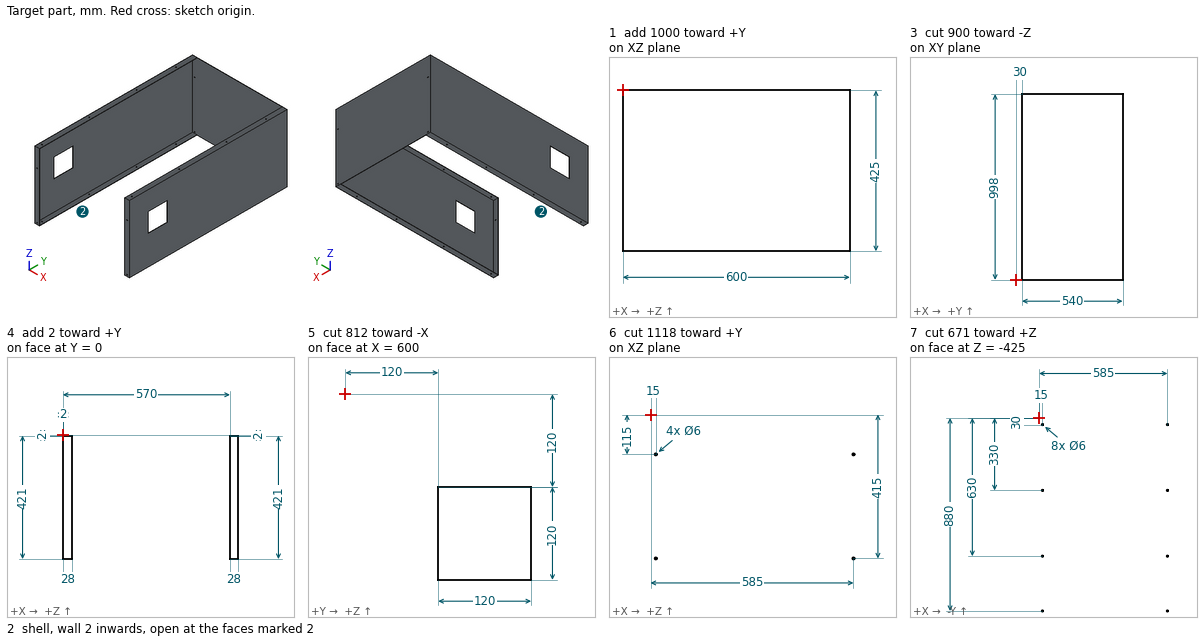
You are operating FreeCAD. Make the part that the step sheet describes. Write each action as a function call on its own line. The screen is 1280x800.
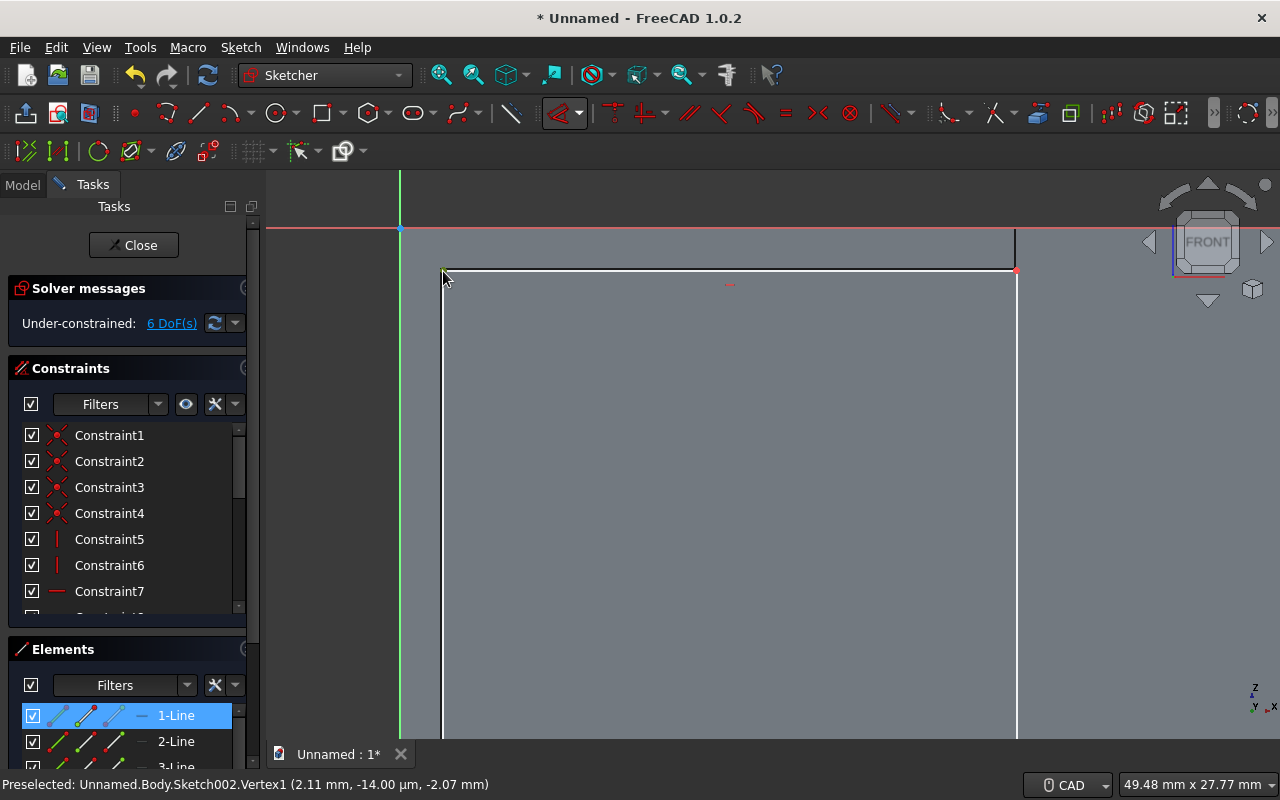
click(582, 114)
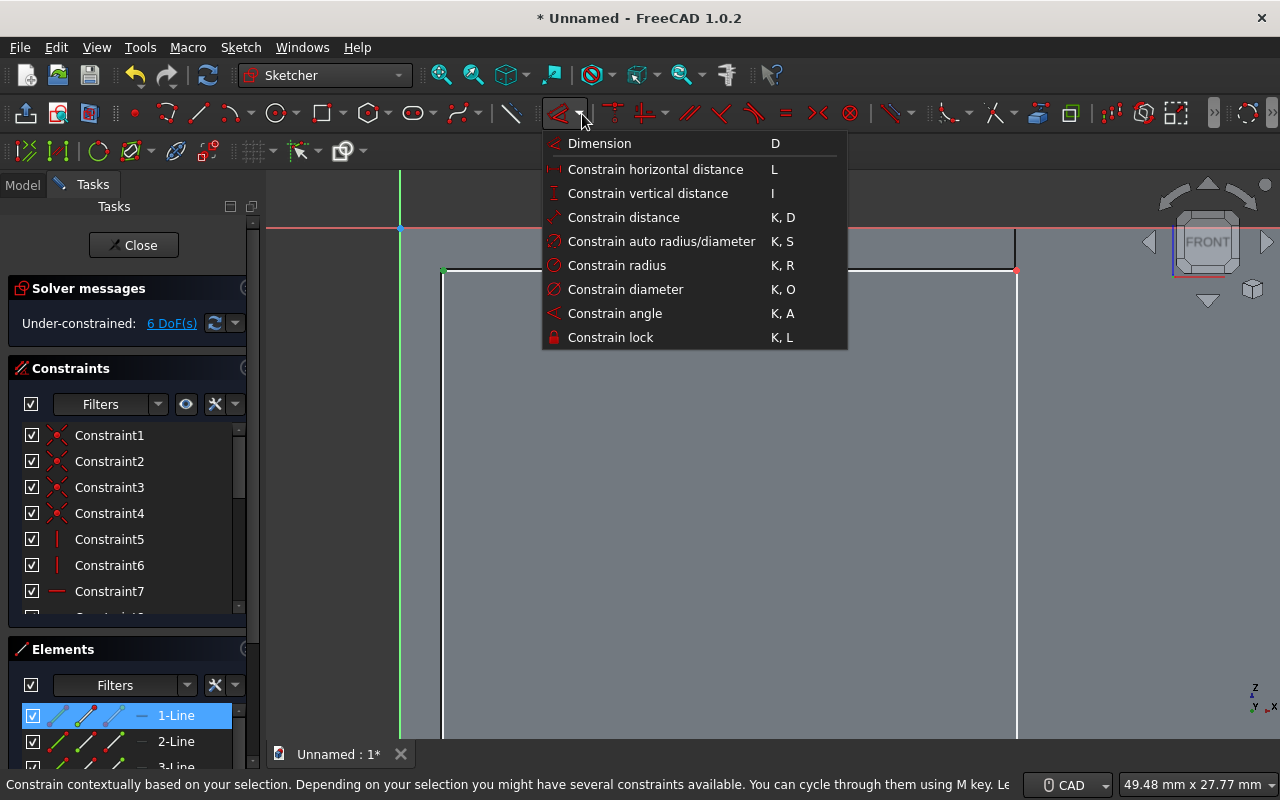
click(695, 169)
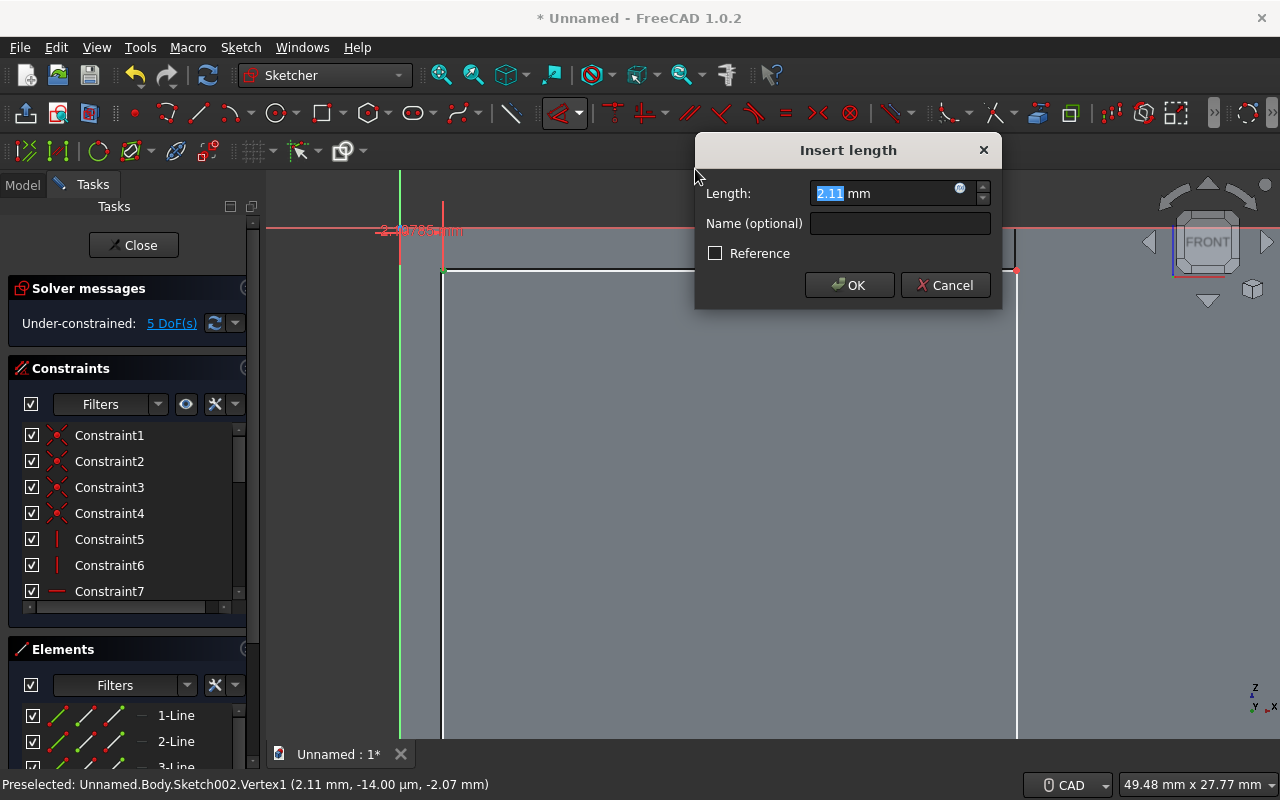
text(2)
key(Return)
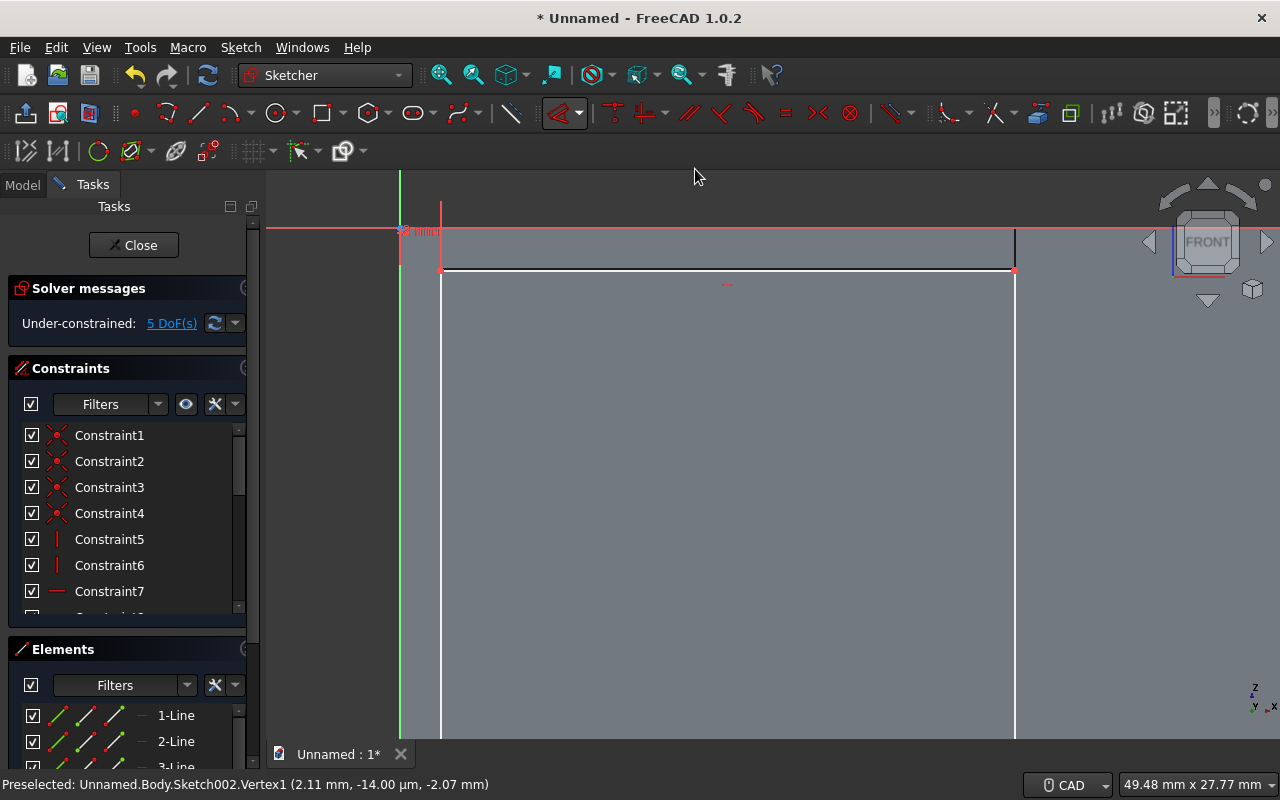
click(441, 271)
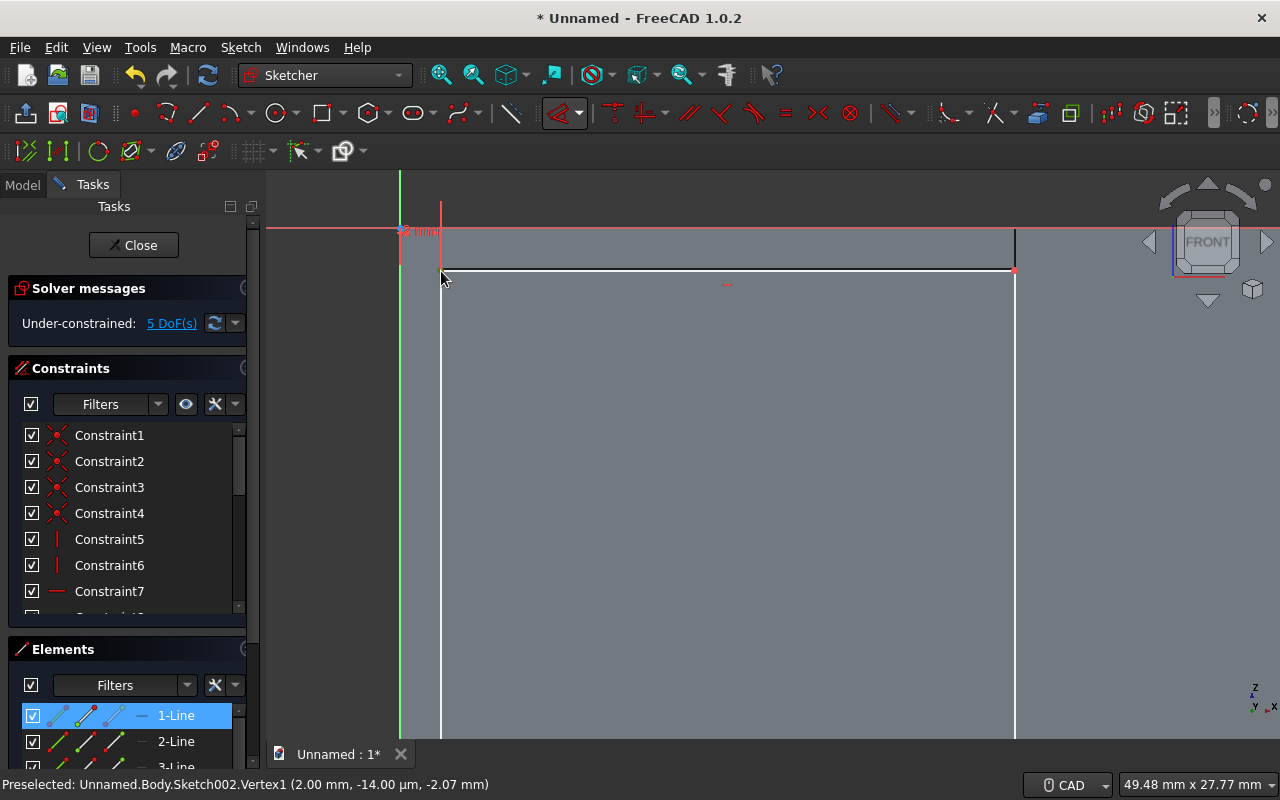
click(582, 114)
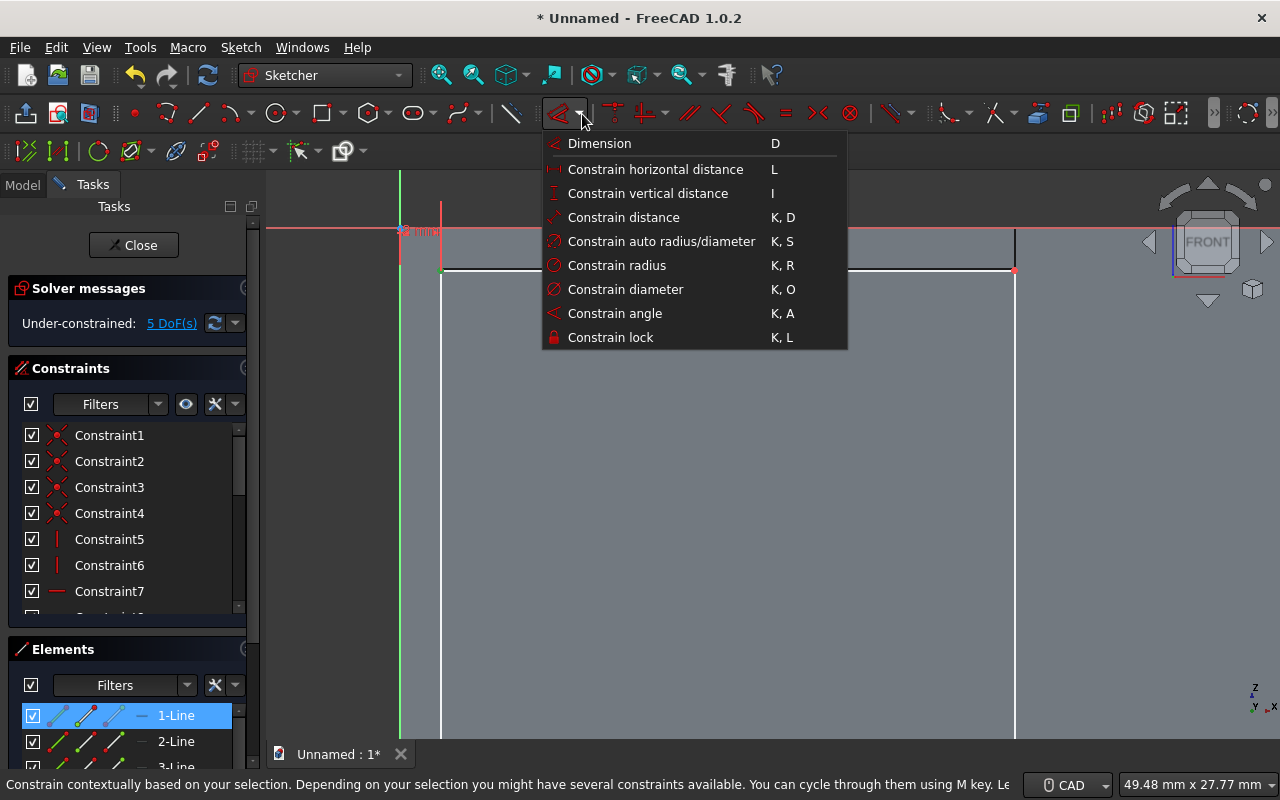
click(695, 193)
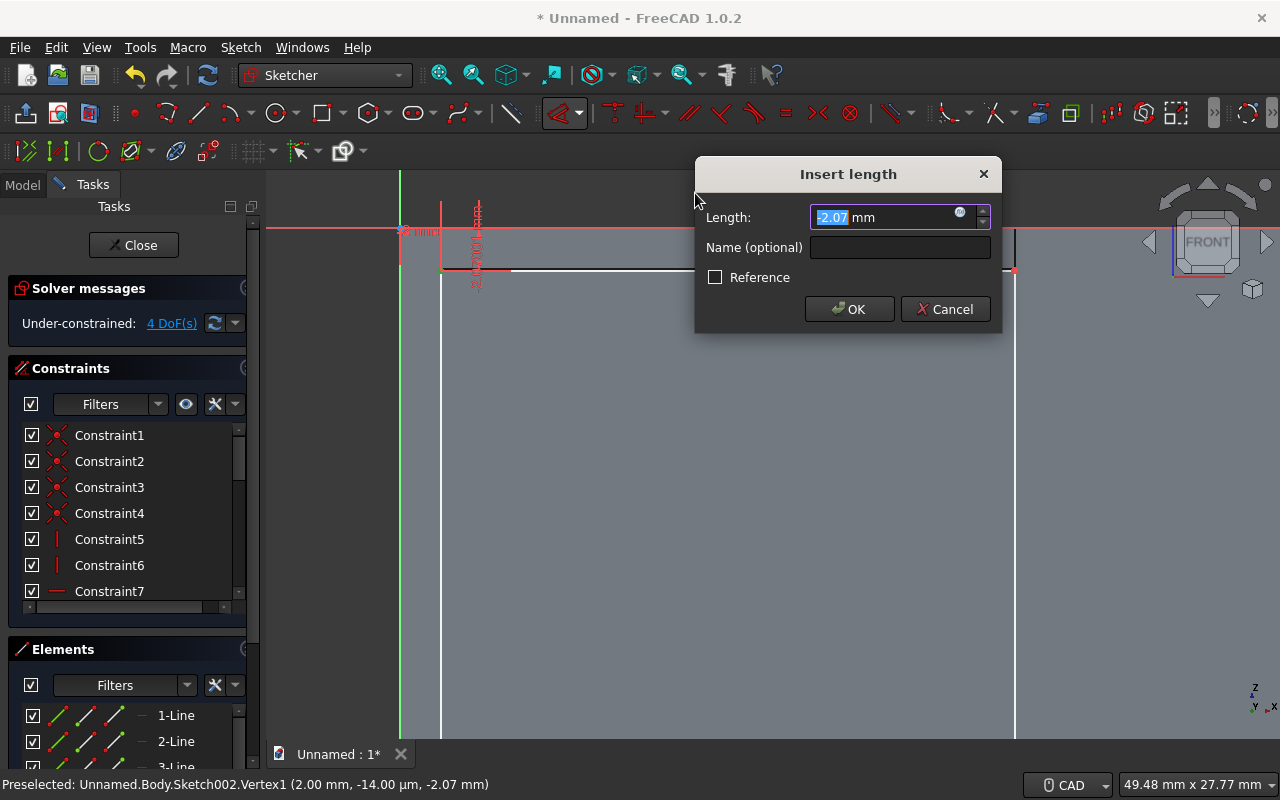
text(-2)
key(Return)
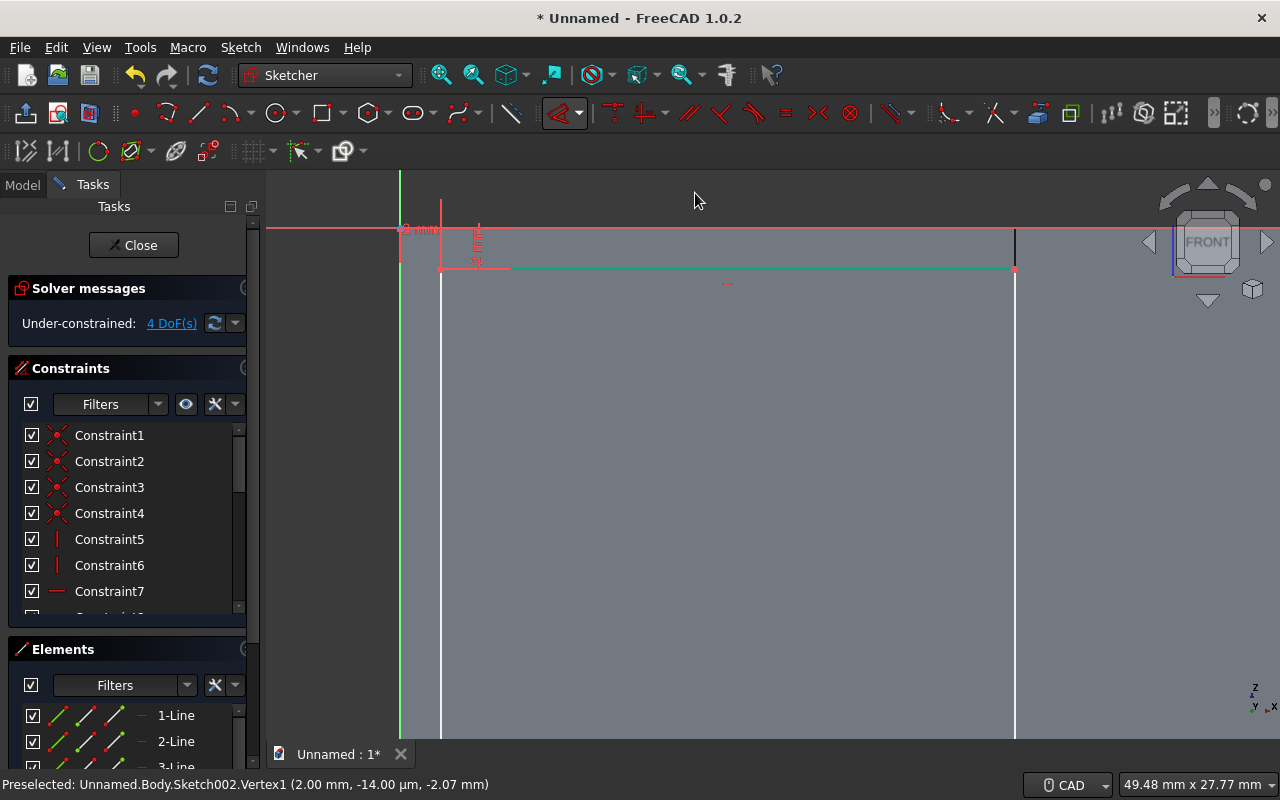
scroll(399, 239, down, 15)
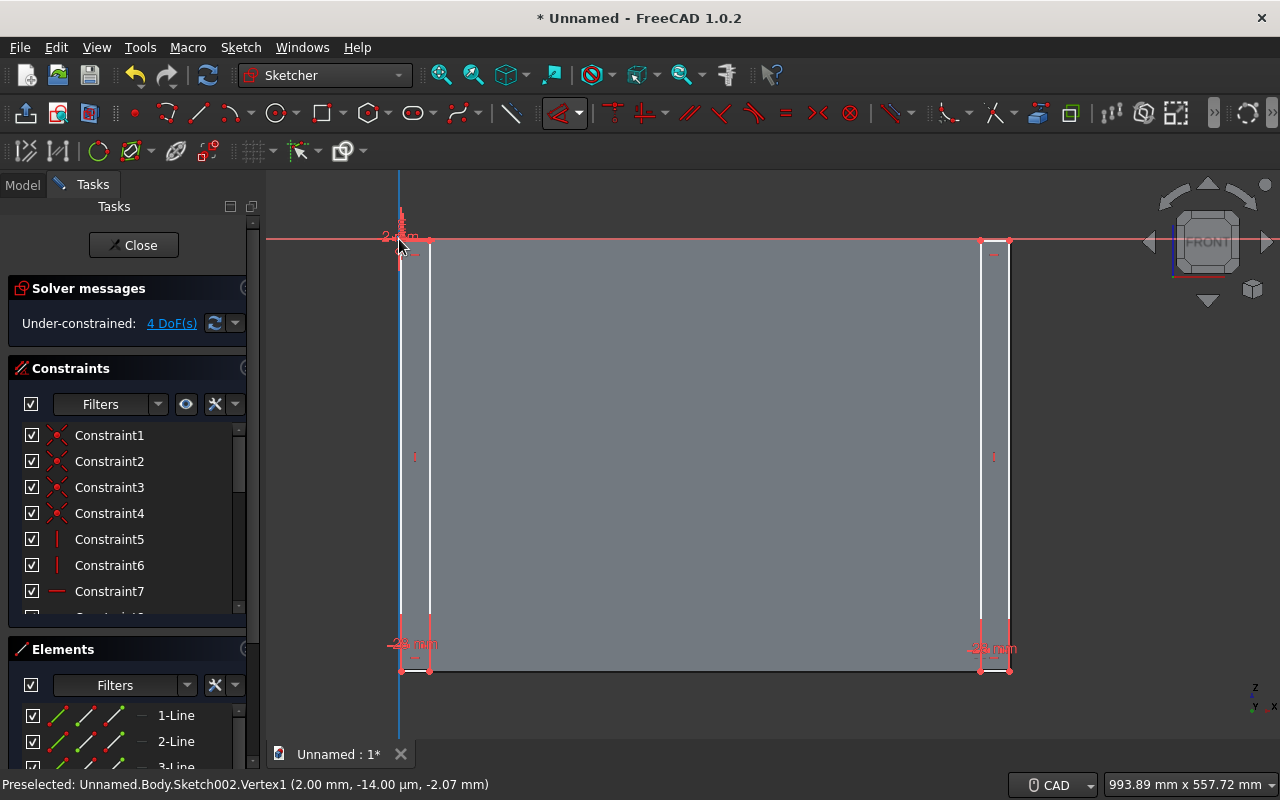
scroll(981, 241, up, 15)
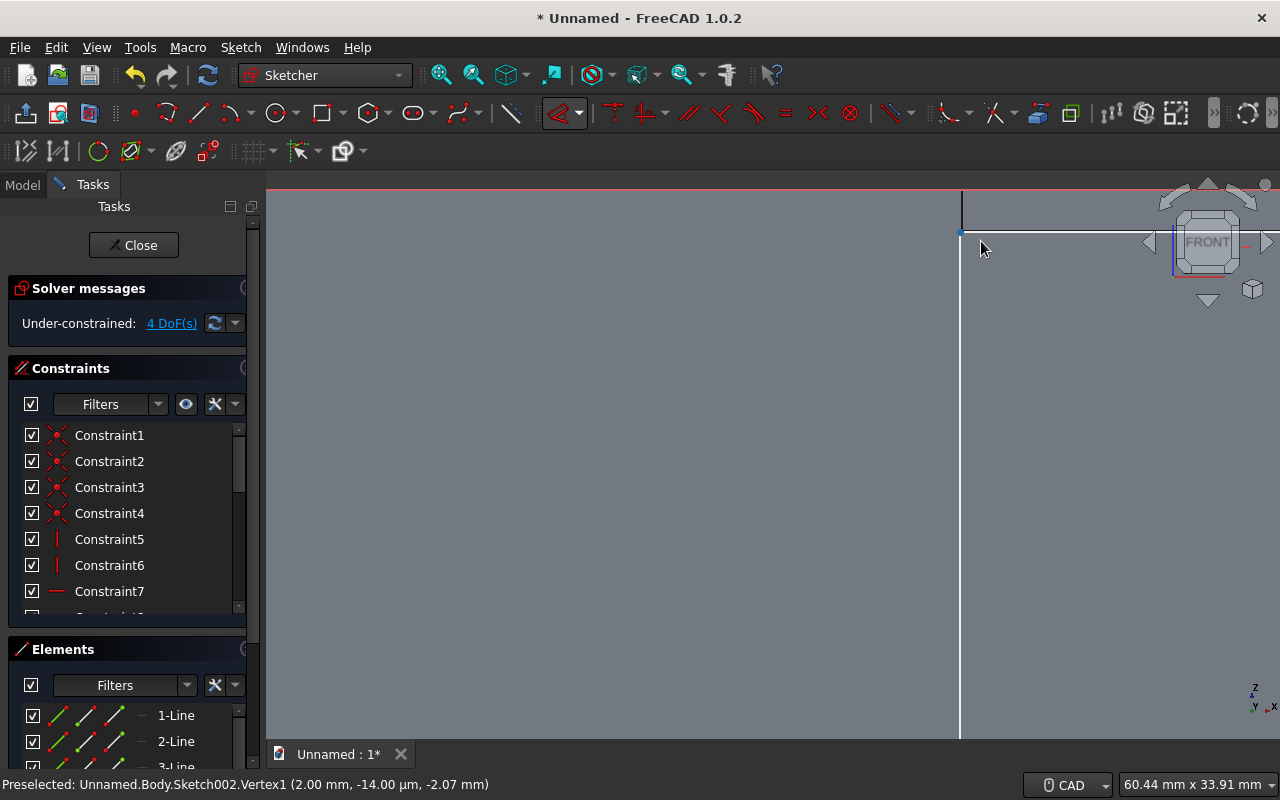
click(960, 232)